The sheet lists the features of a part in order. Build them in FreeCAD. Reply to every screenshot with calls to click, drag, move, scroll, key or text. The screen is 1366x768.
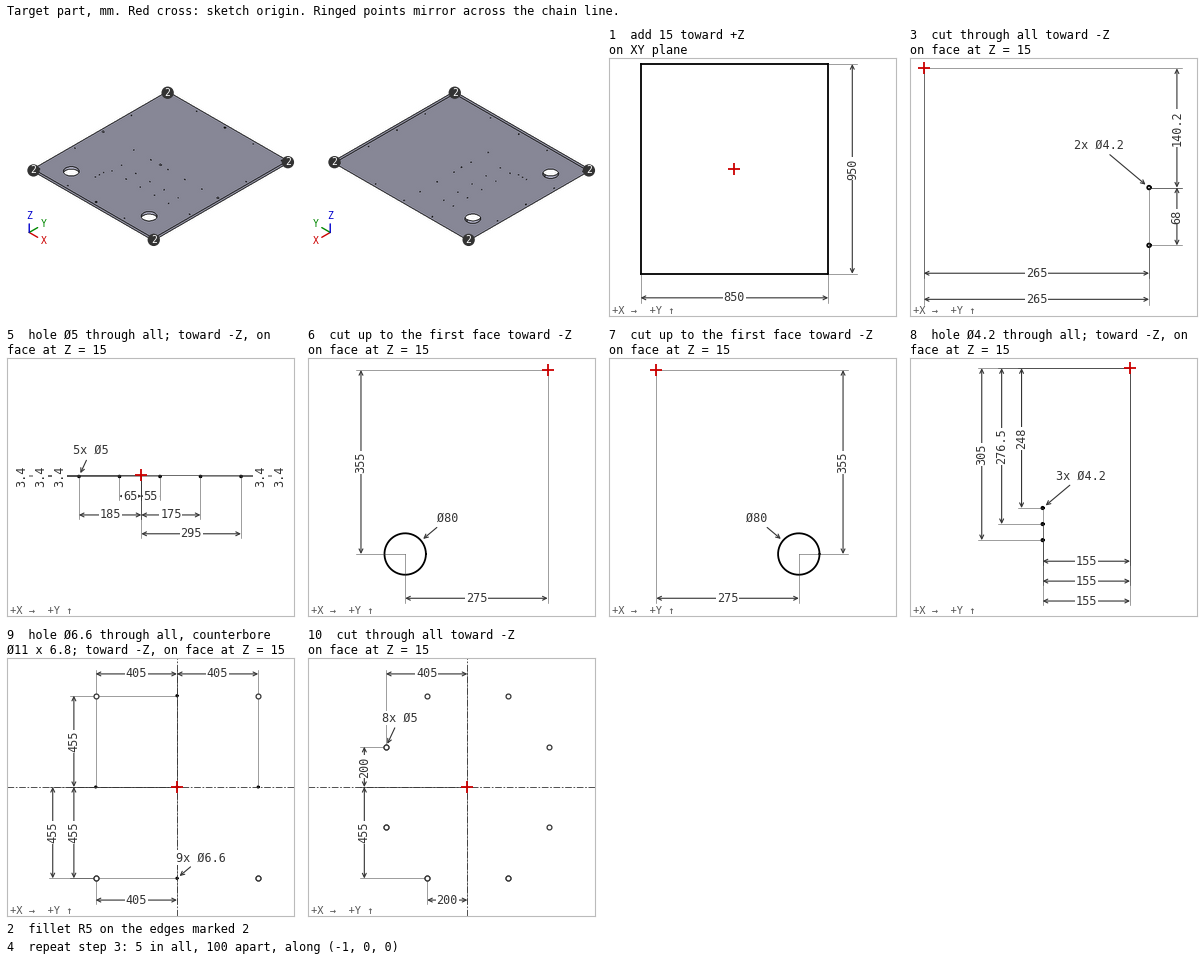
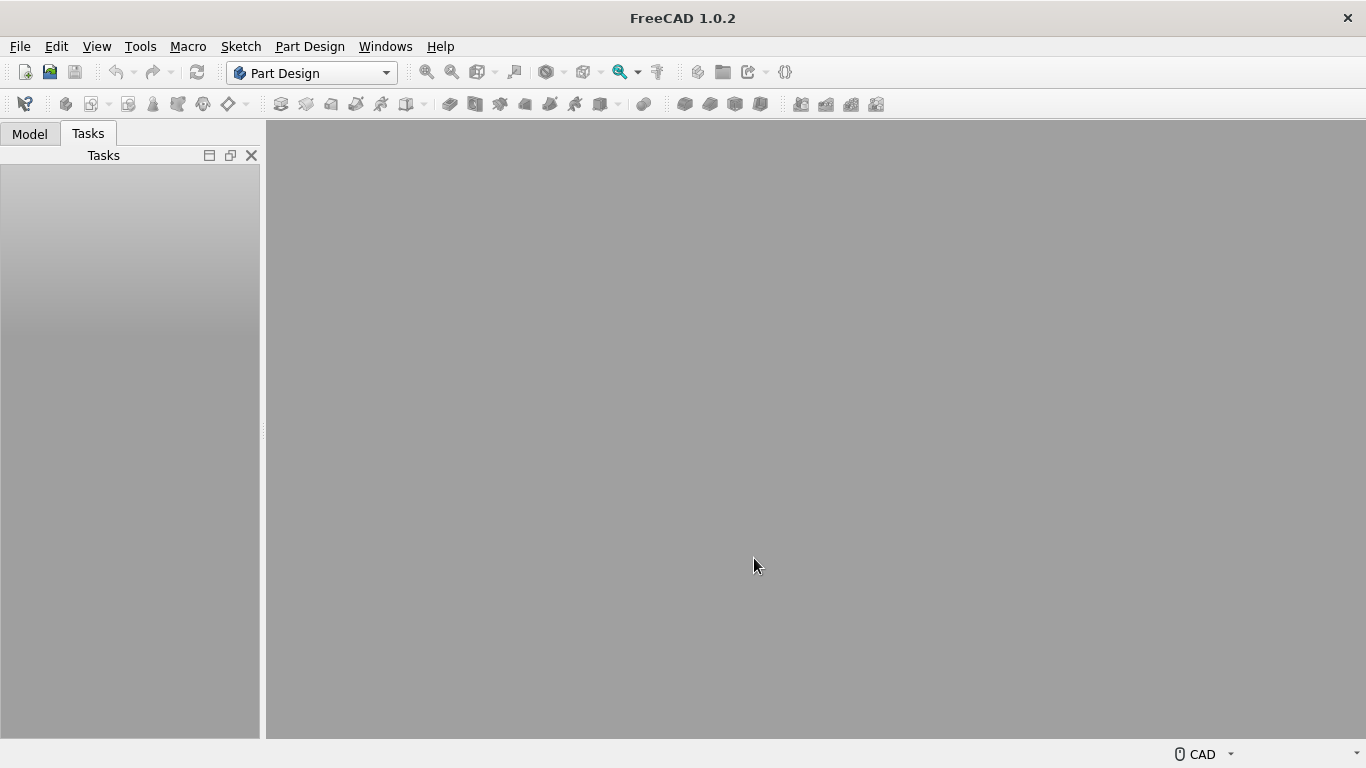
click(25, 72)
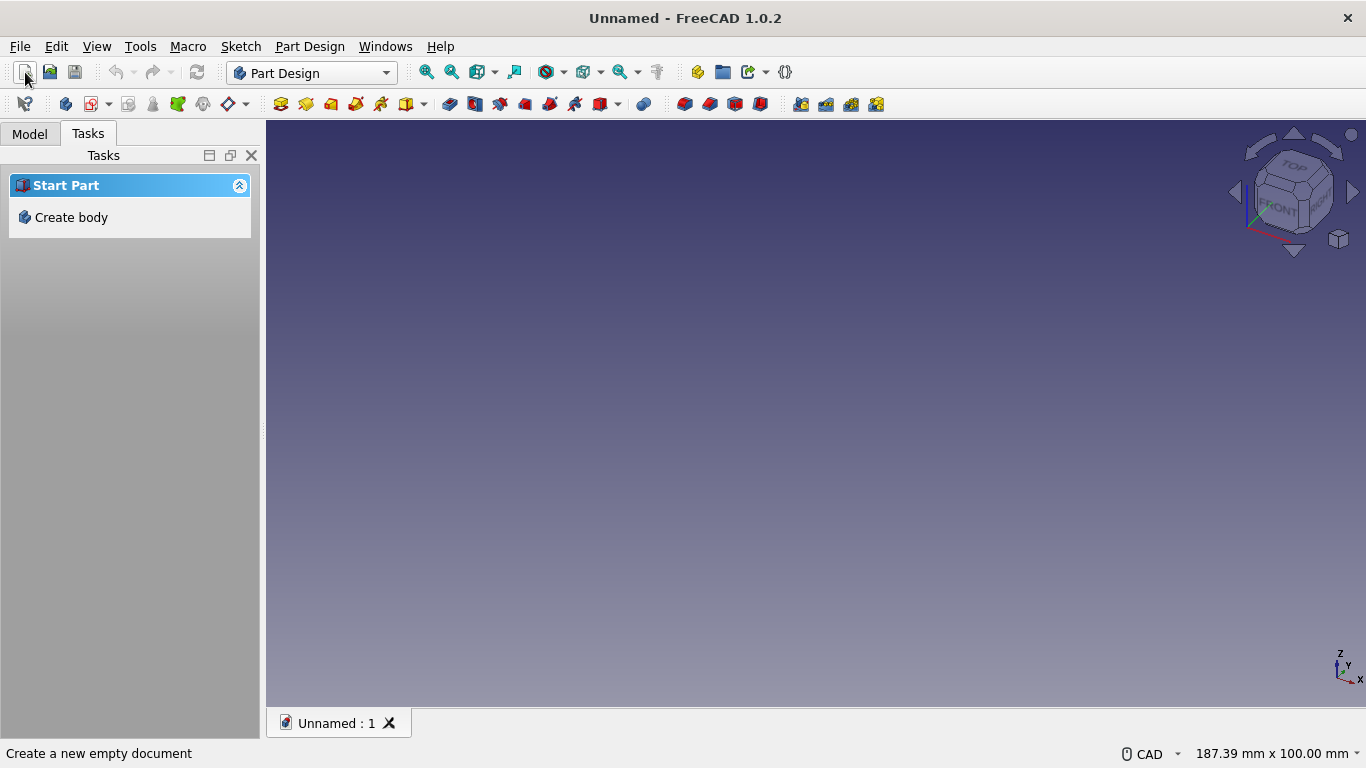
click(90, 104)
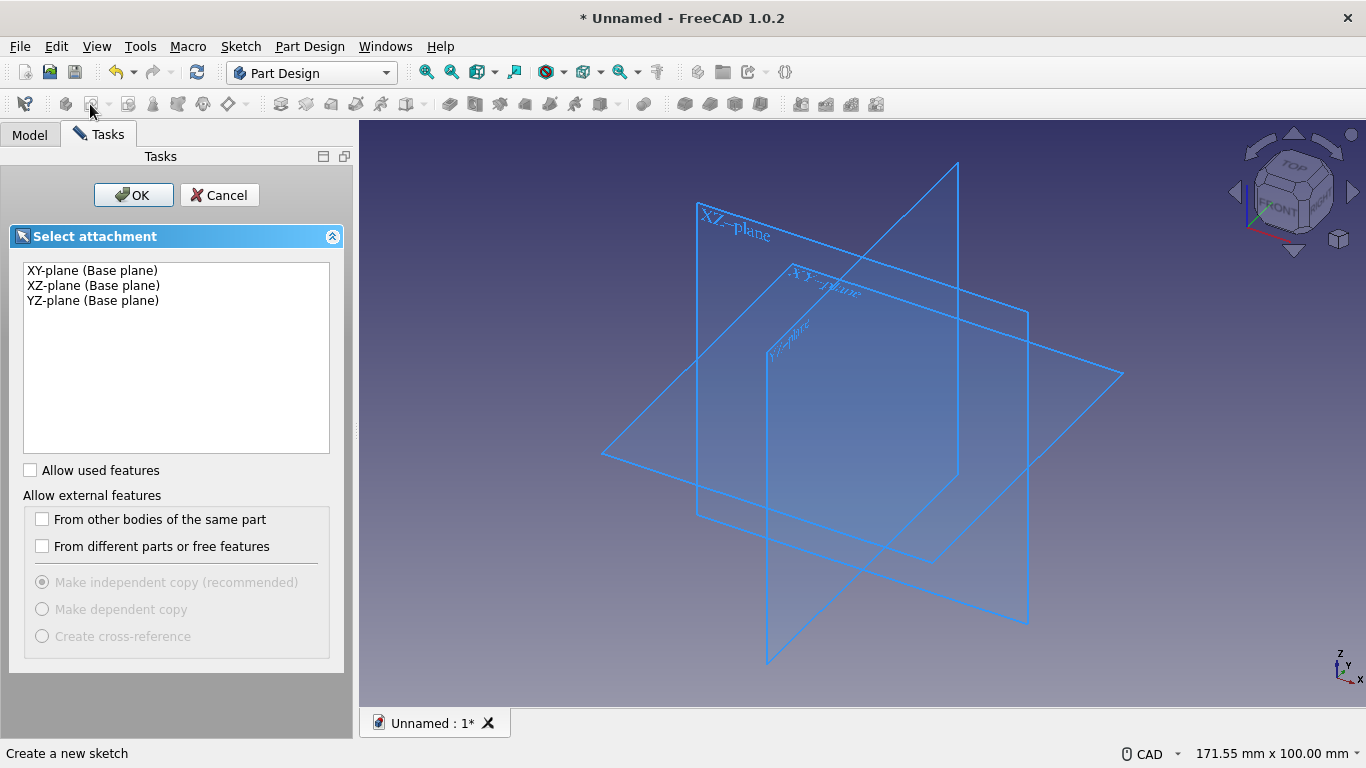
click(84, 270)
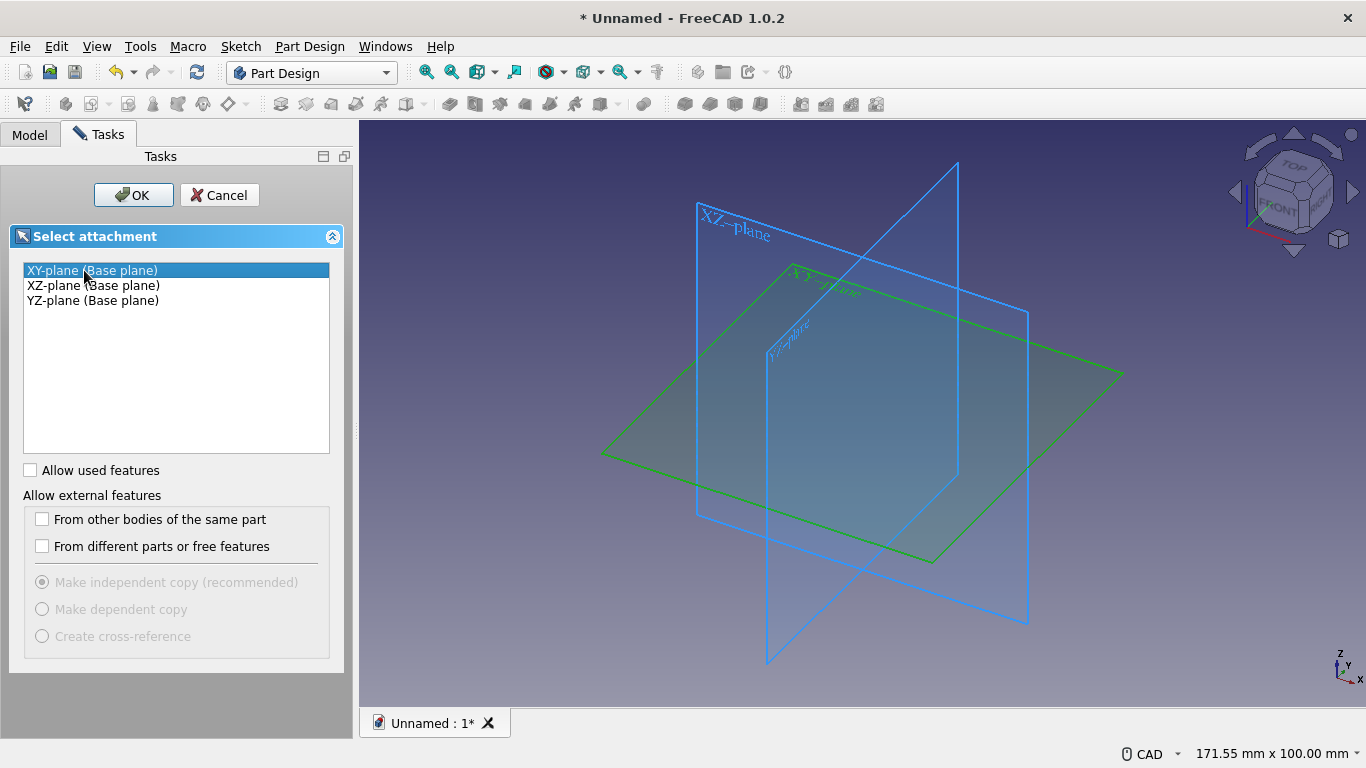
click(134, 195)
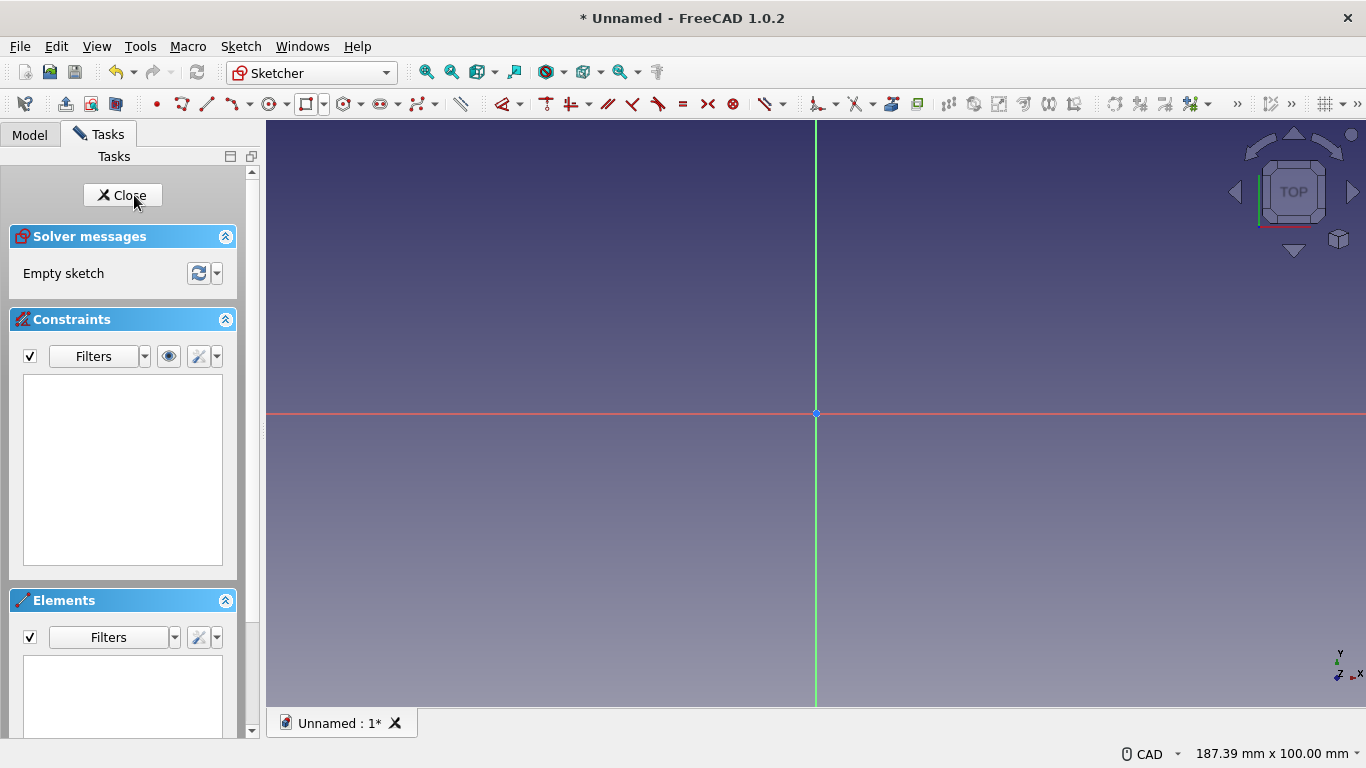
scroll(743, 414, down, 14)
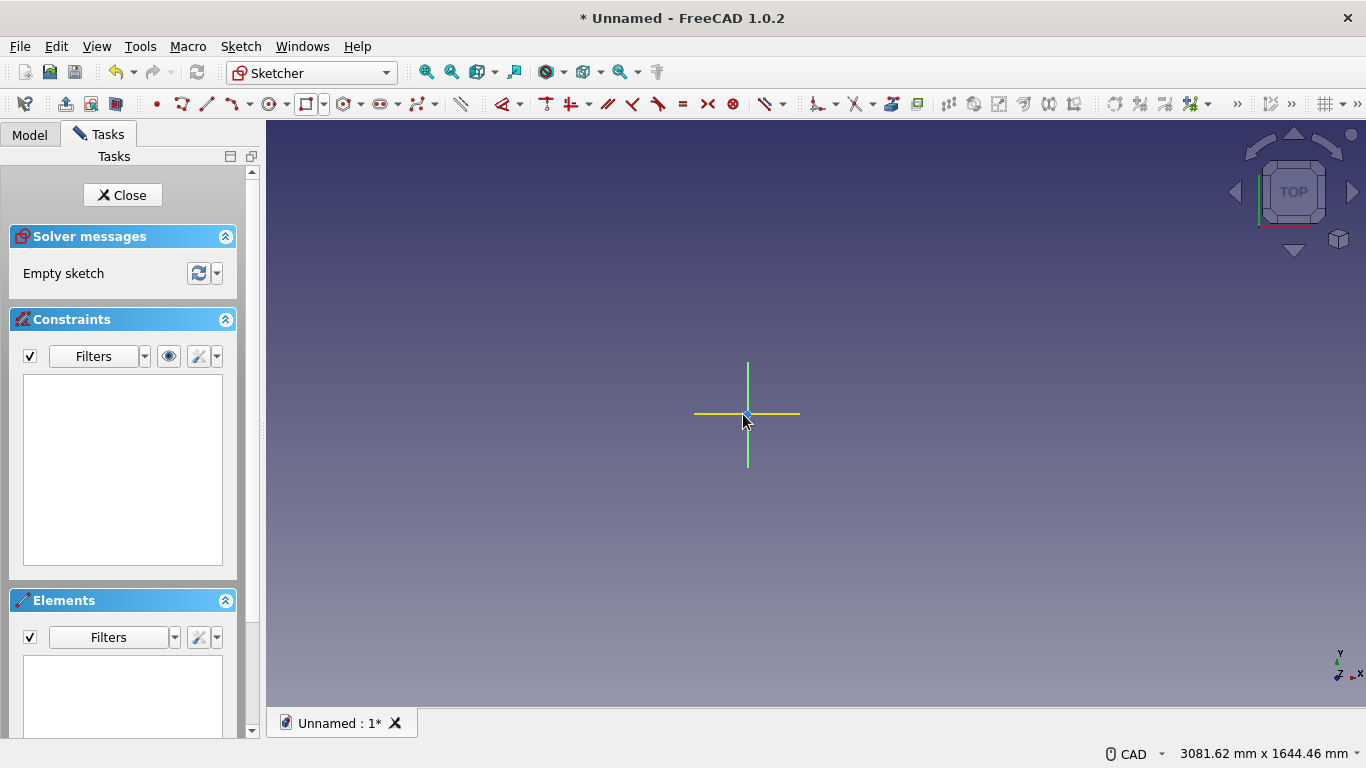
click(324, 104)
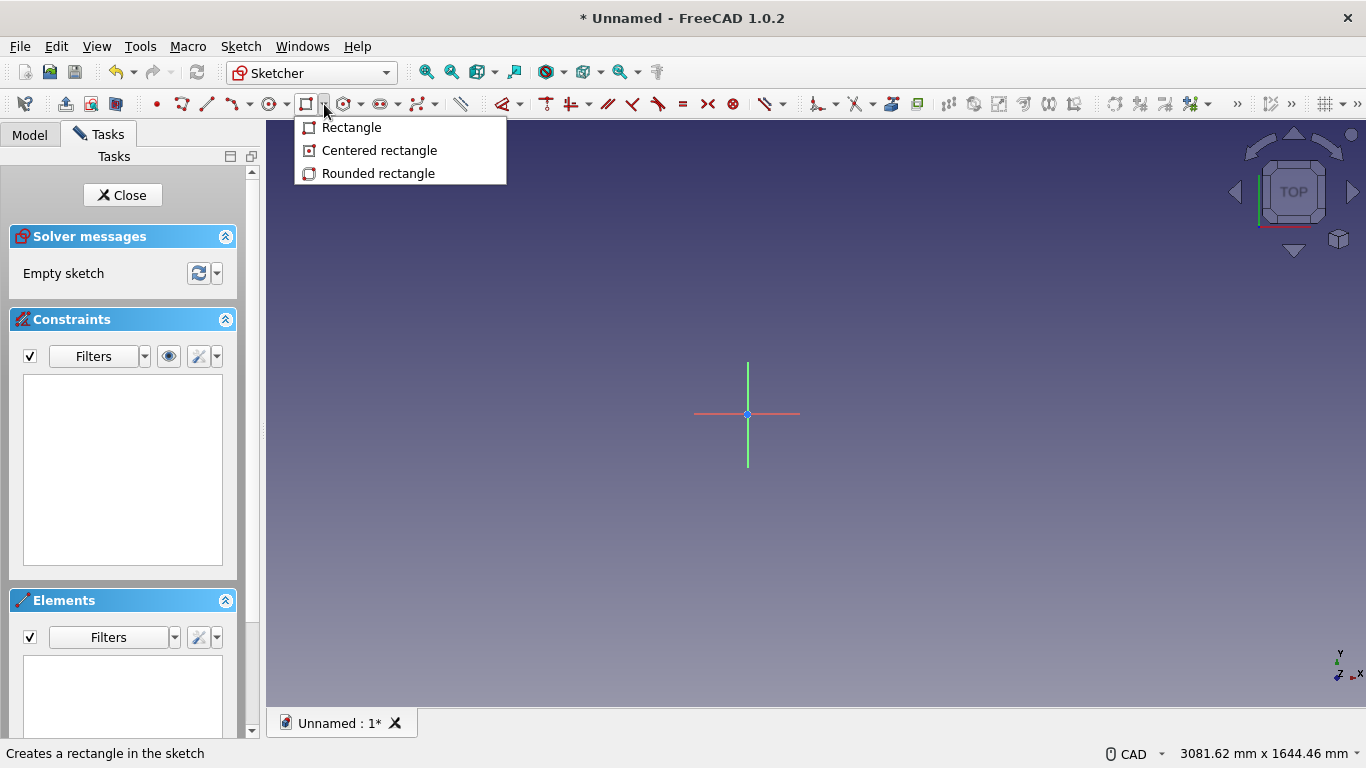
click(400, 150)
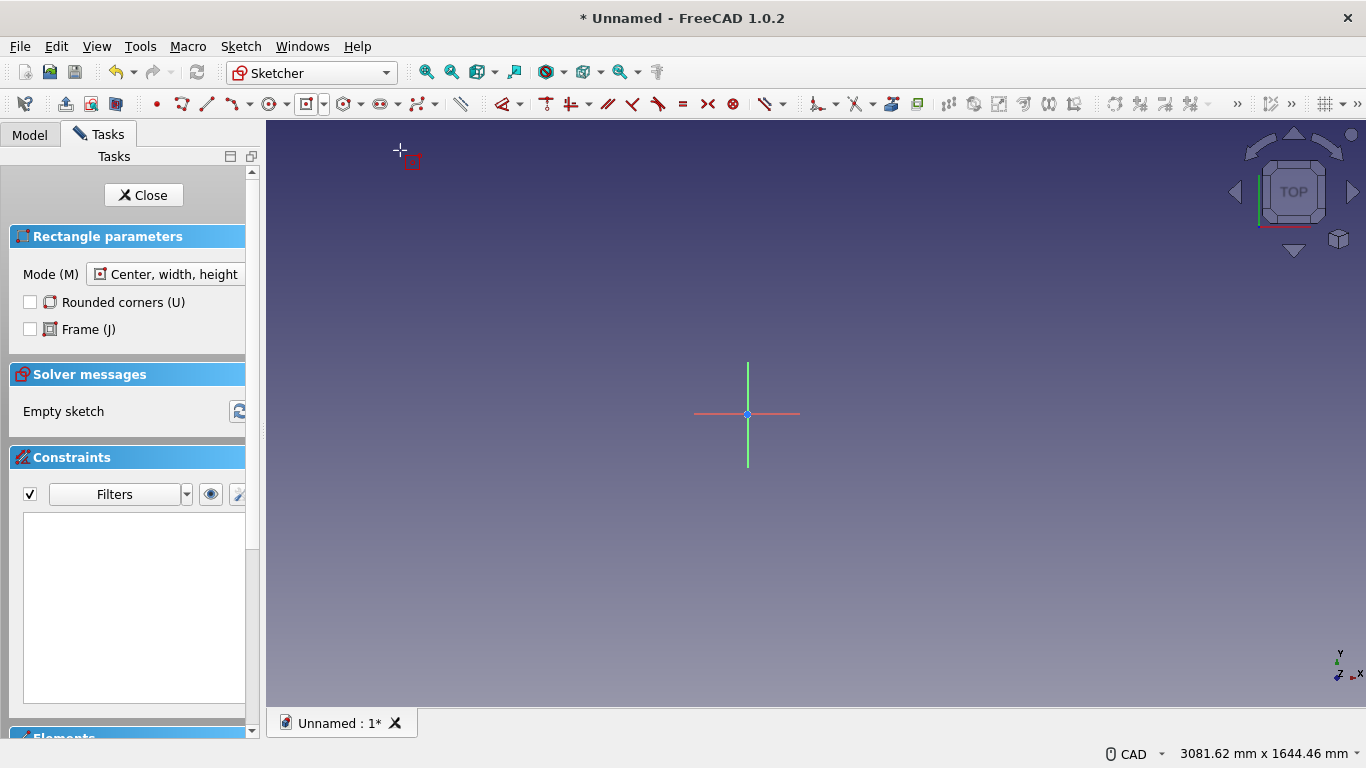
click(748, 414)
move(900, 245)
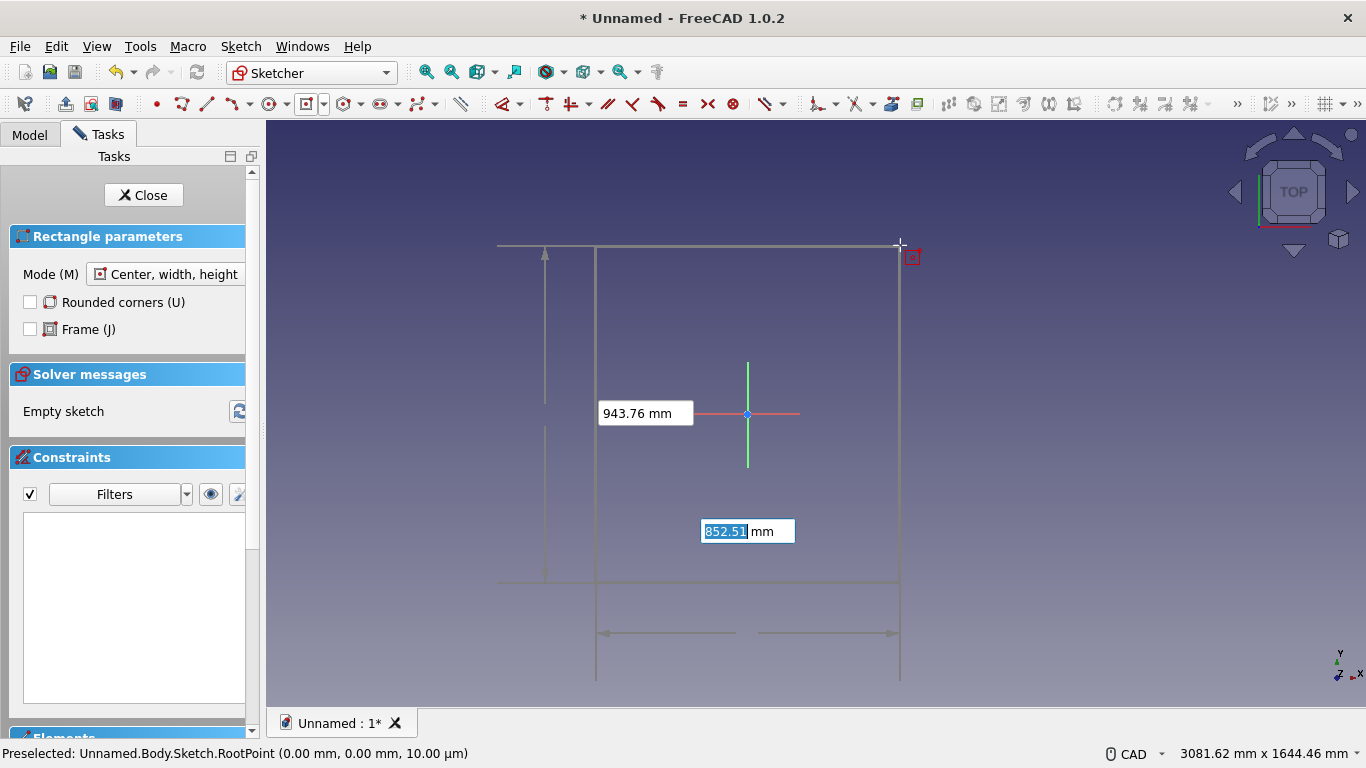
text(850)
key(Tab)
text(950)
key(Return)
key(Escape)